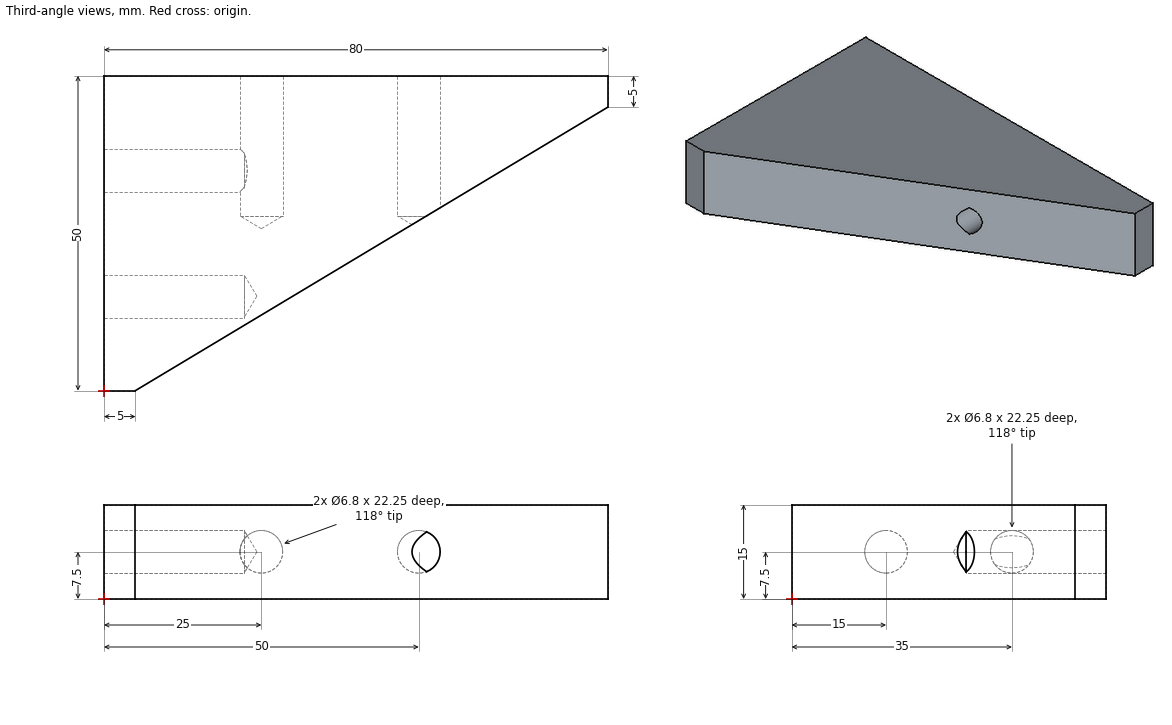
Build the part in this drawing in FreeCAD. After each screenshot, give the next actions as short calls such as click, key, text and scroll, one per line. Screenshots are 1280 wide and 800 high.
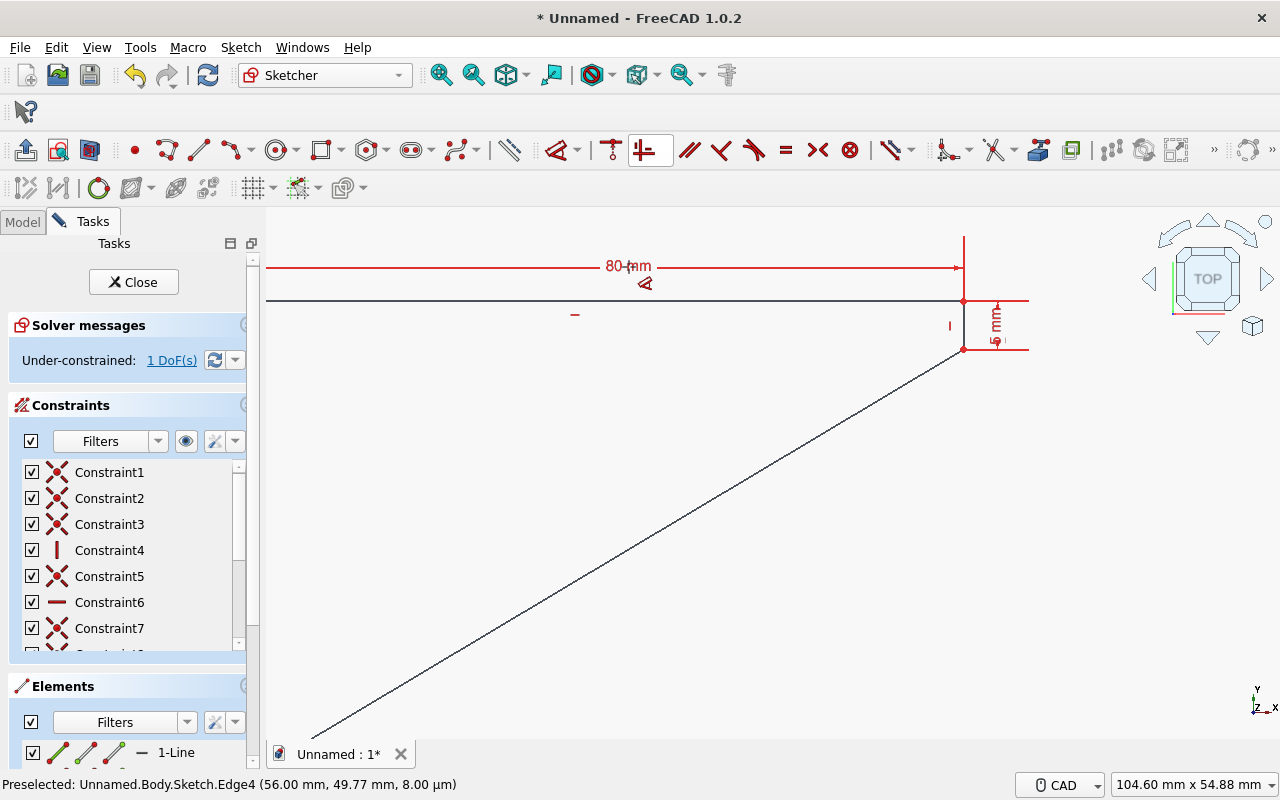
scroll(966, 334, down, 2)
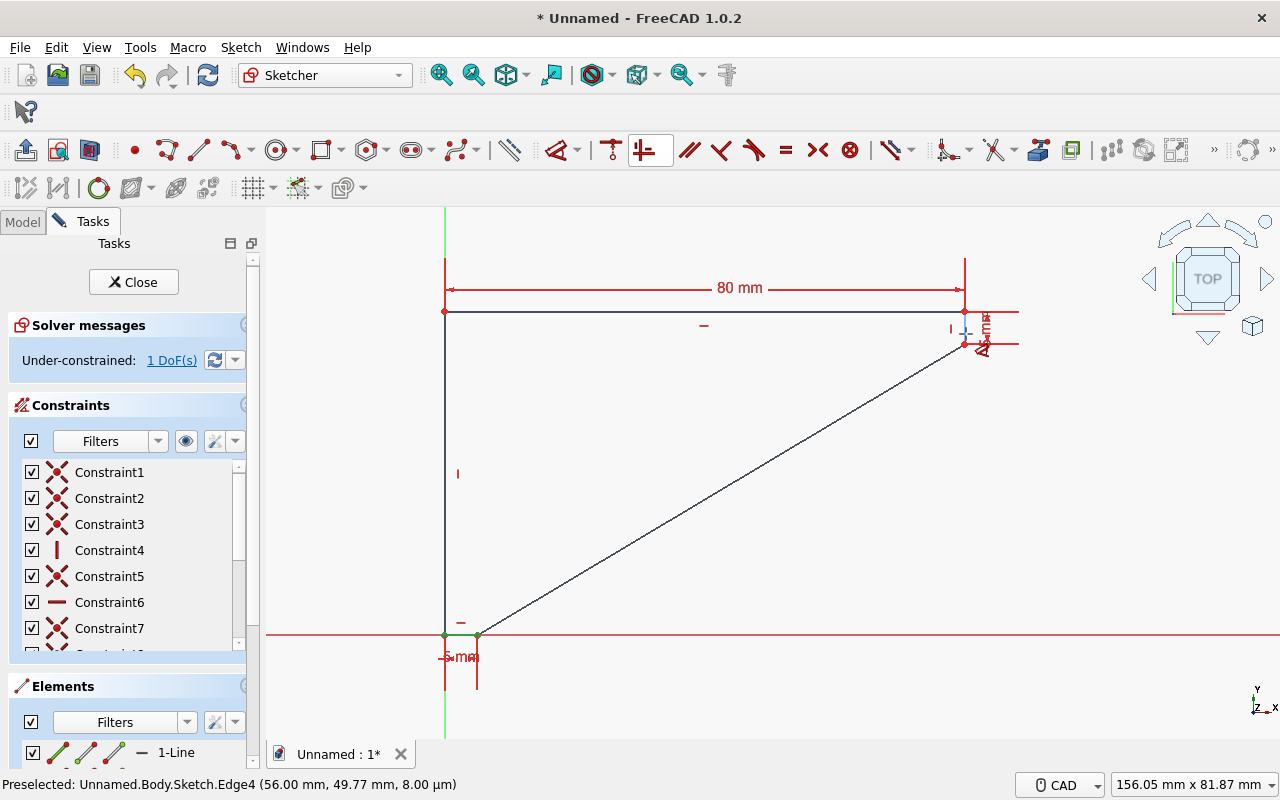
click(445, 409)
click(411, 474)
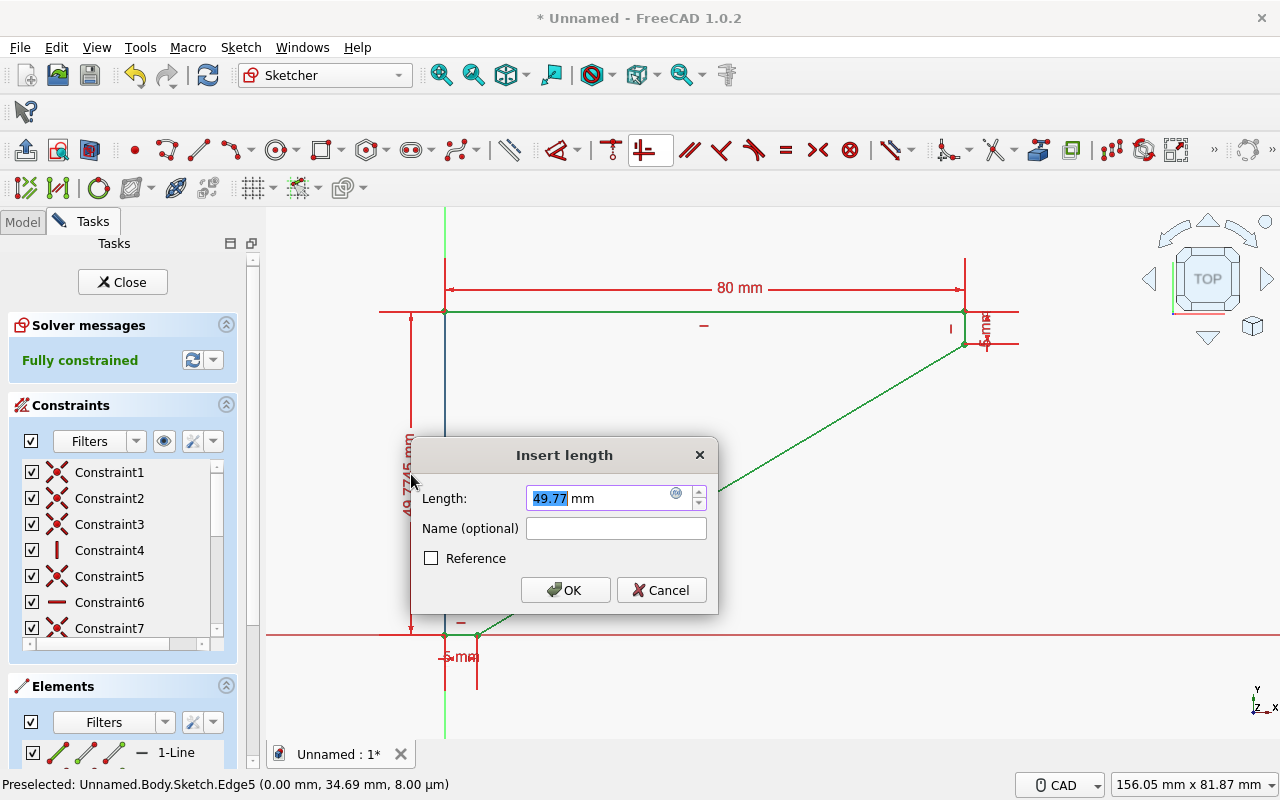
text(50)
key(Return)
key(Escape)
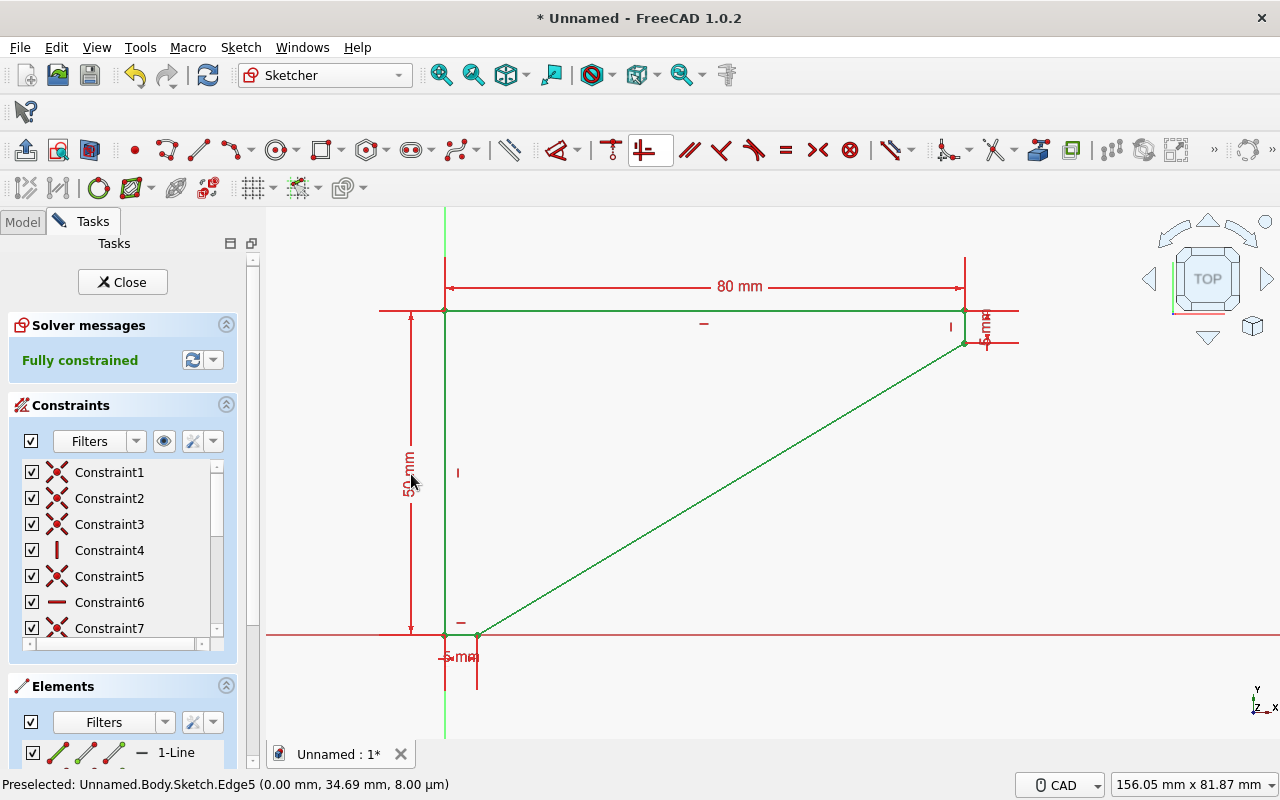
click(123, 282)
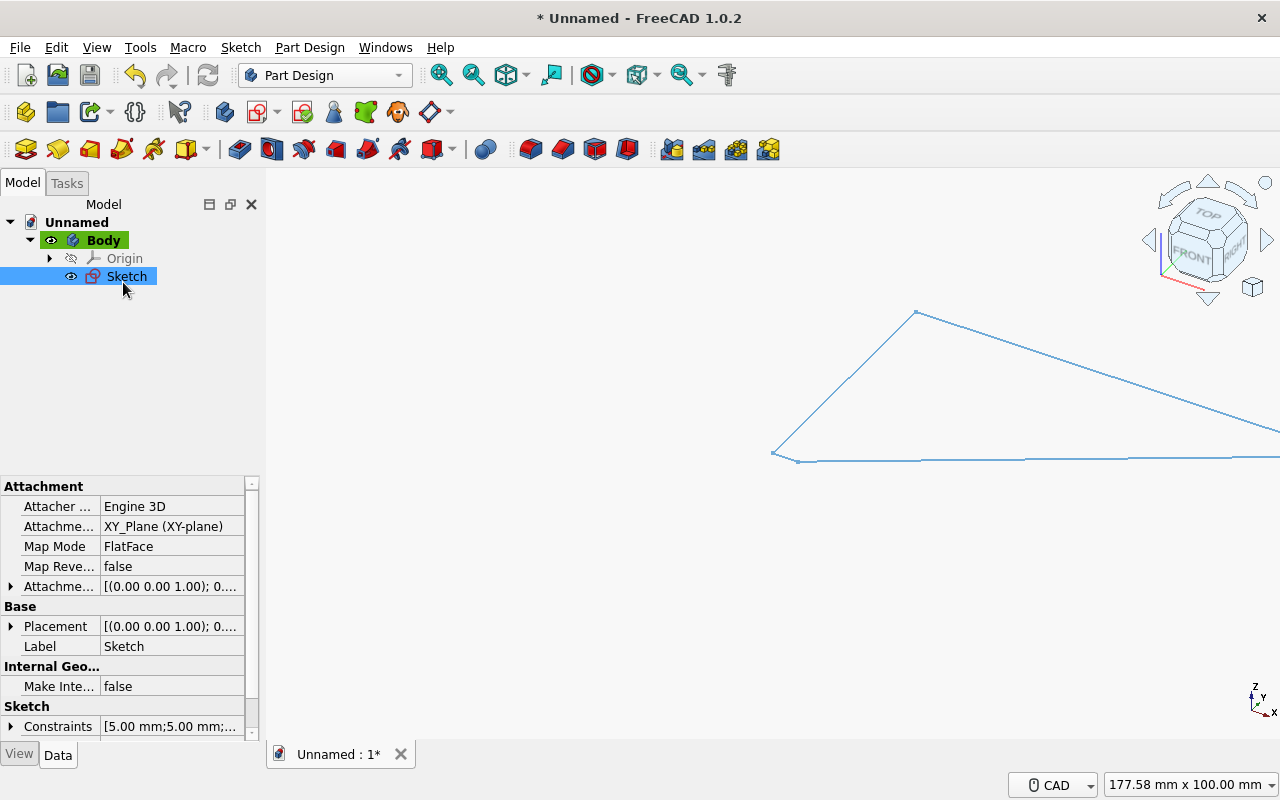
click(26, 150)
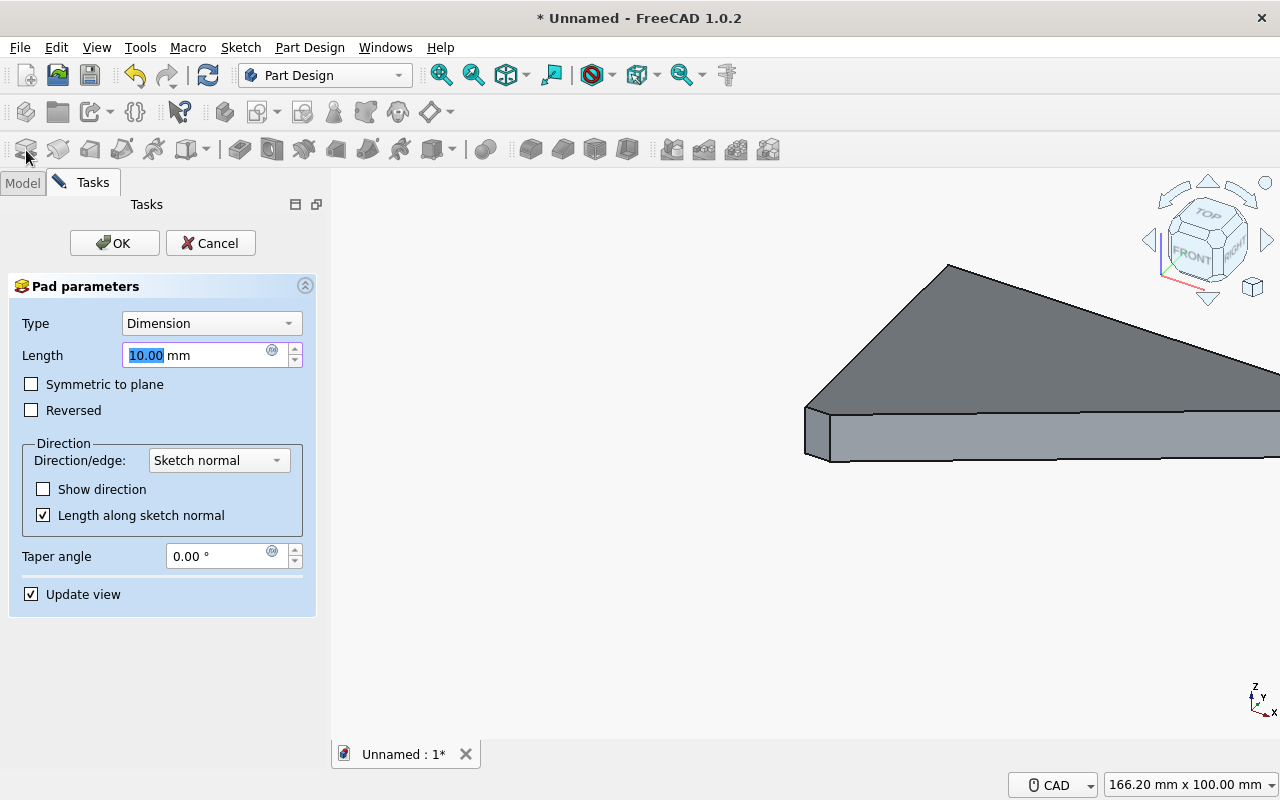
text(15)
key(Tab)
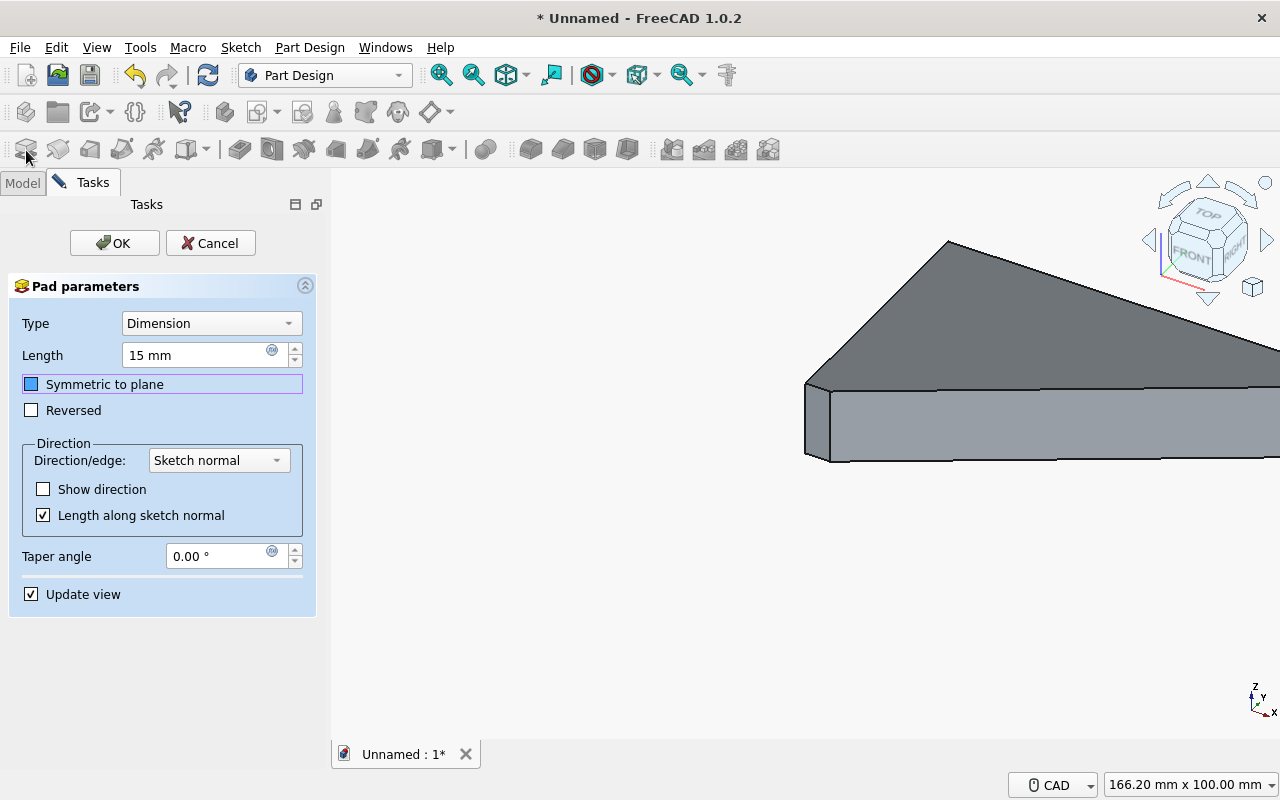
click(115, 243)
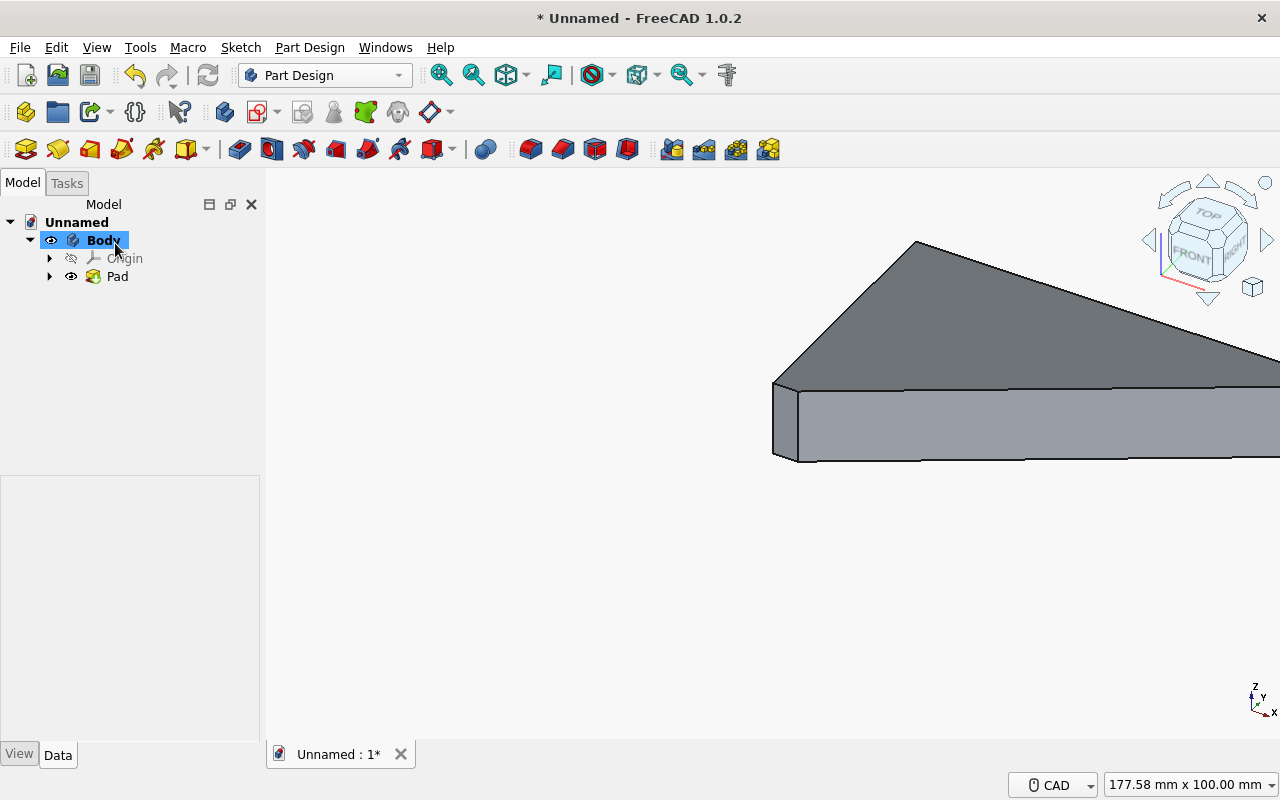
click(442, 76)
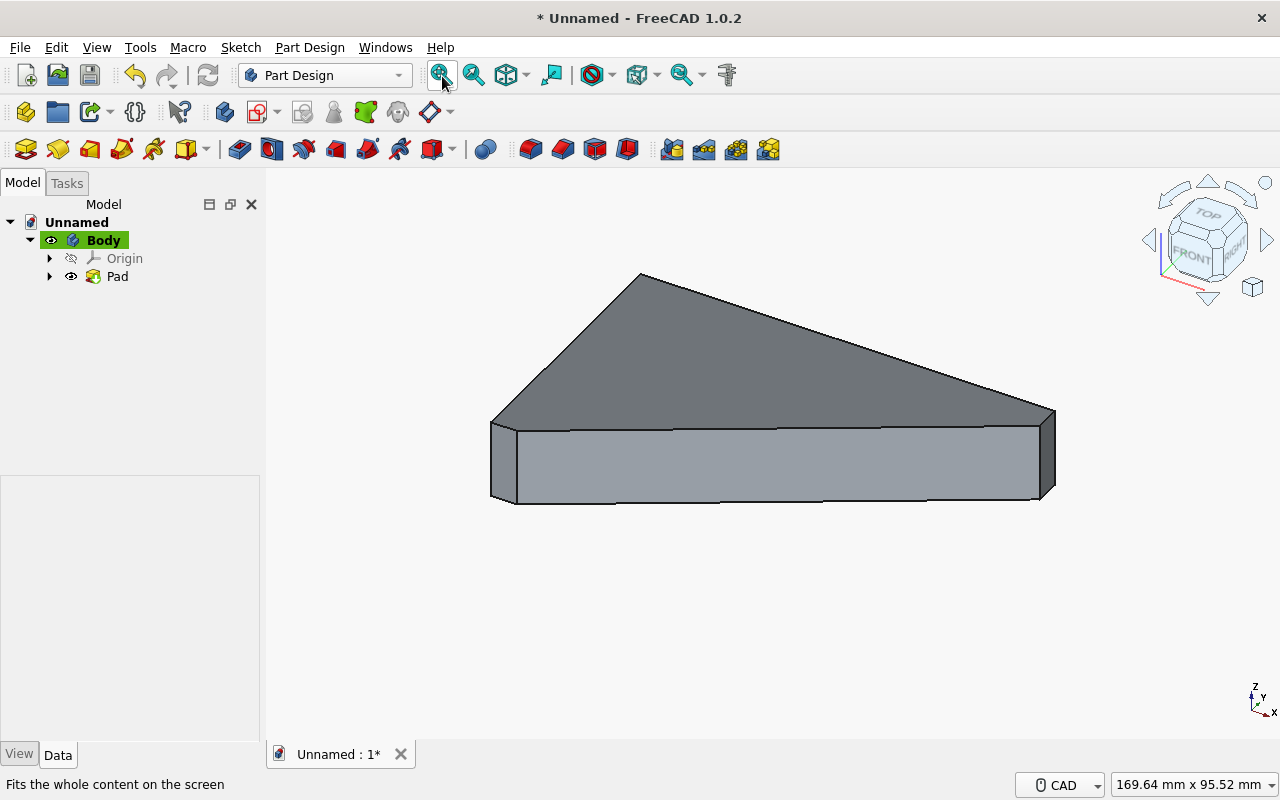
key(4)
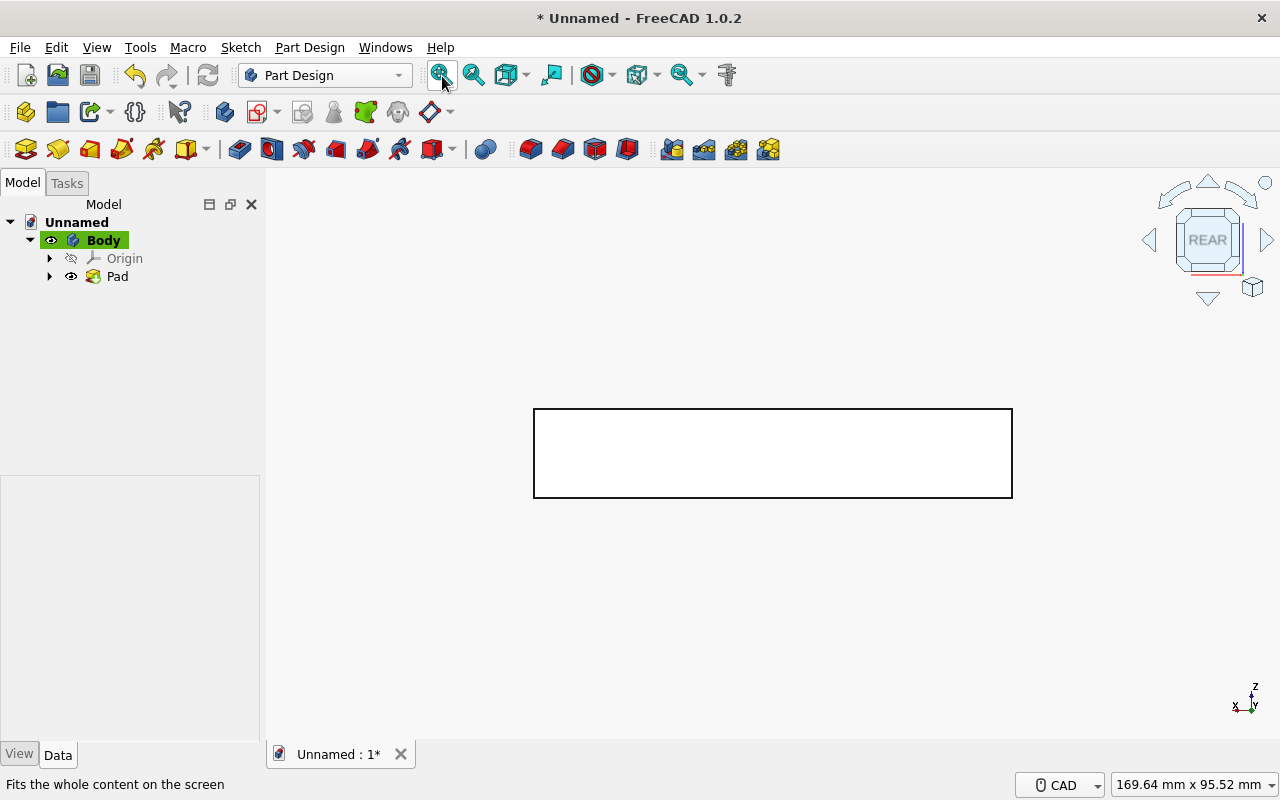
click(636, 452)